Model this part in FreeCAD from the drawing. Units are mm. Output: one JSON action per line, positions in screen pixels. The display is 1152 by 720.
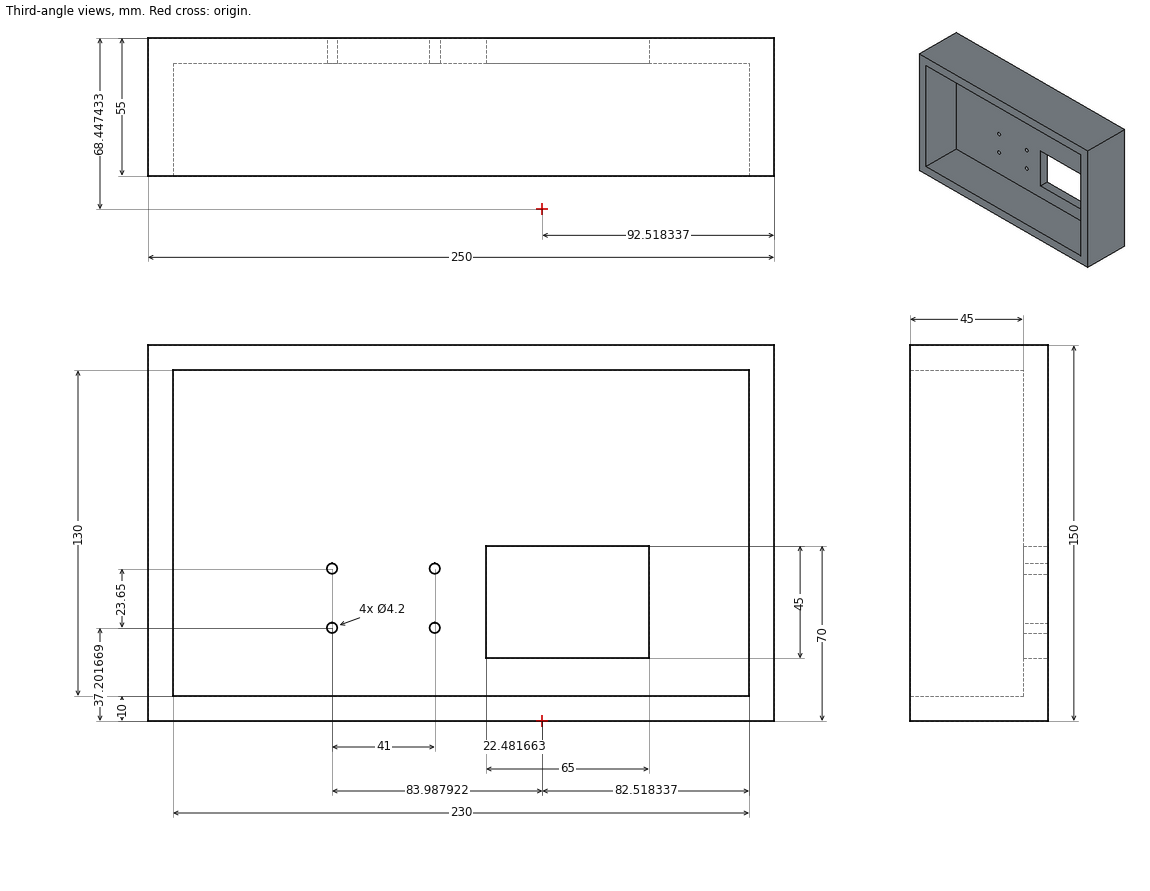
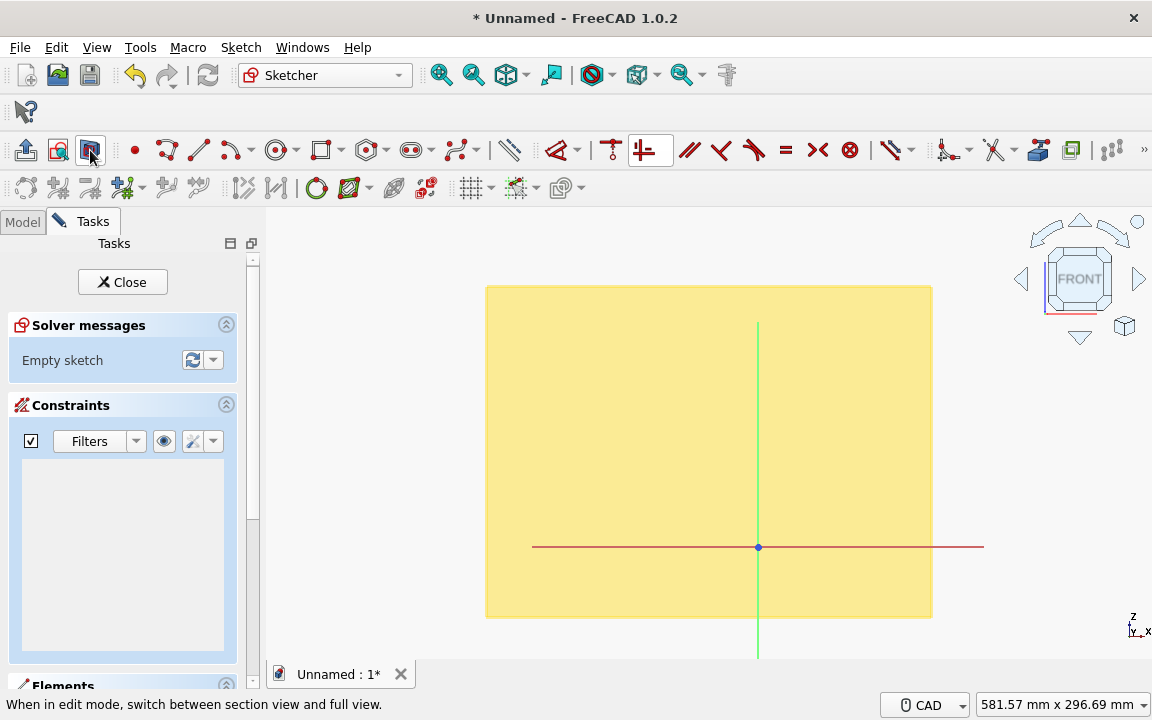
{"action": "scroll", "coordinate": [723, 538], "scroll_direction": "up", "scroll_amount": 5}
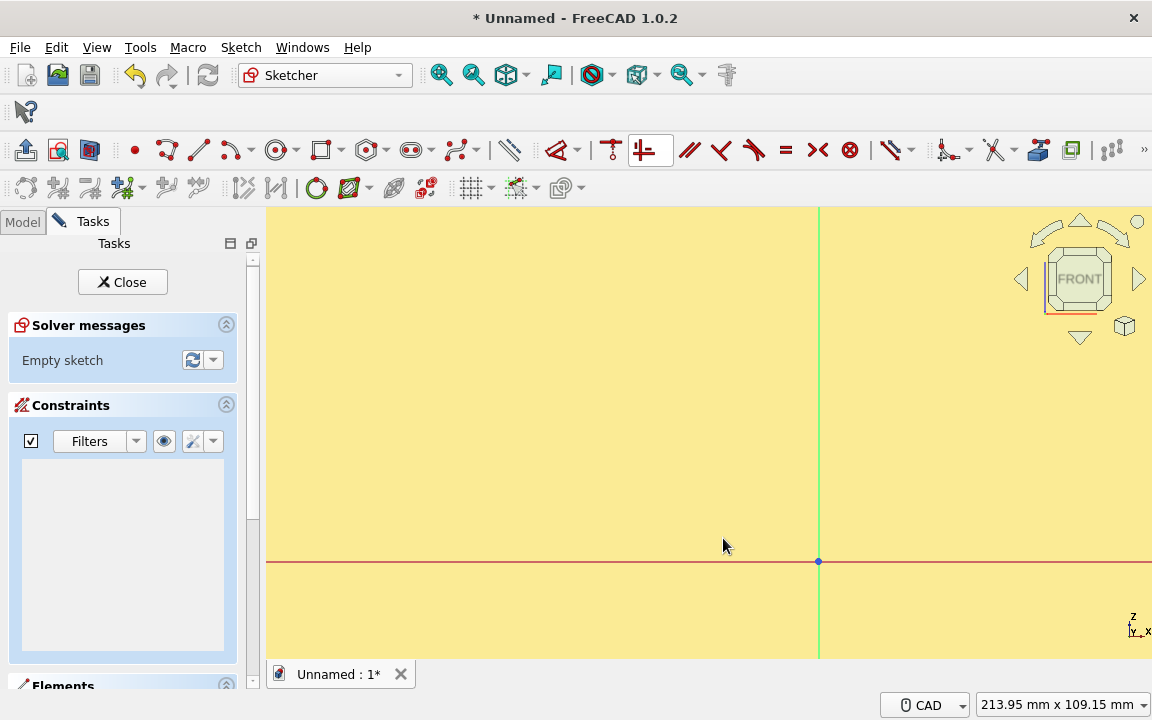
{"action": "left_click", "coordinate": [276, 150]}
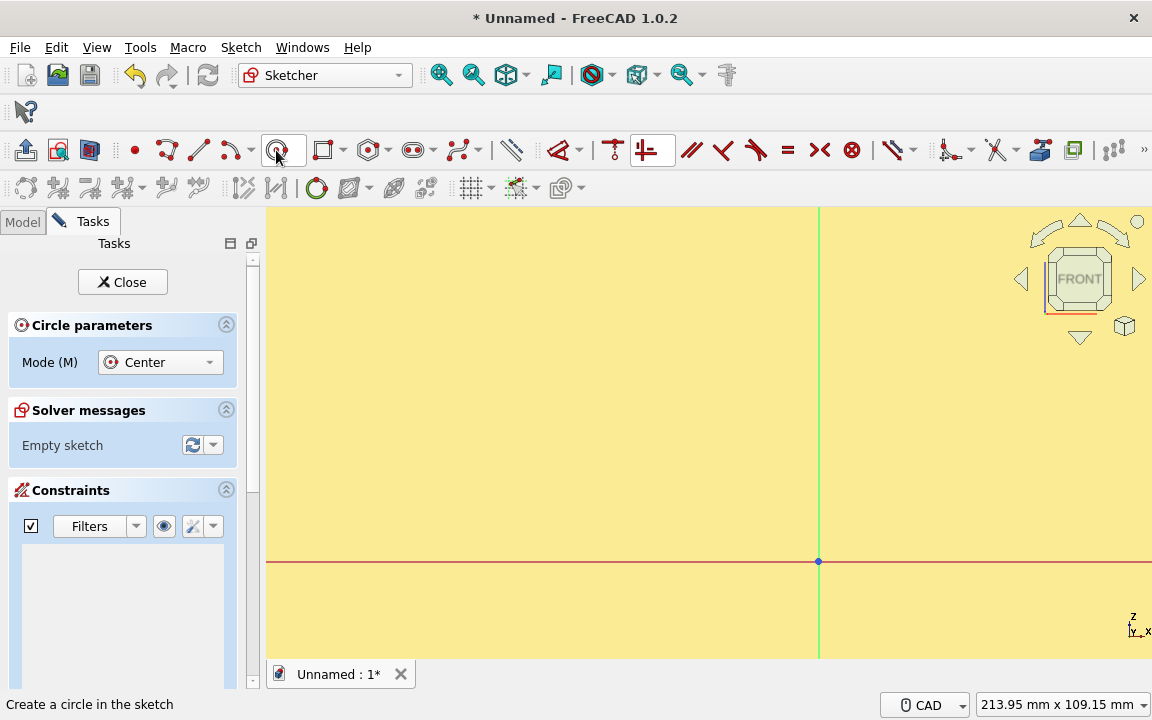
{"action": "scroll", "coordinate": [471, 408], "scroll_direction": "up", "scroll_amount": 5}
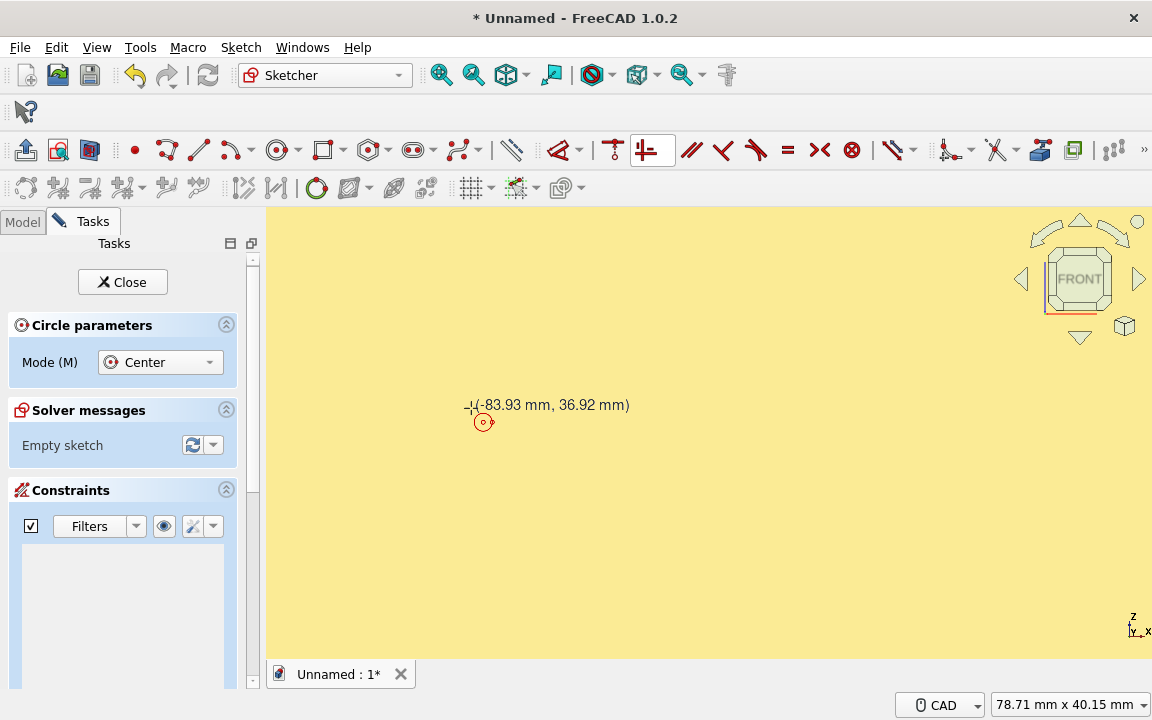
{"action": "left_click", "coordinate": [470, 407]}
{"action": "left_click", "coordinate": [487, 390]}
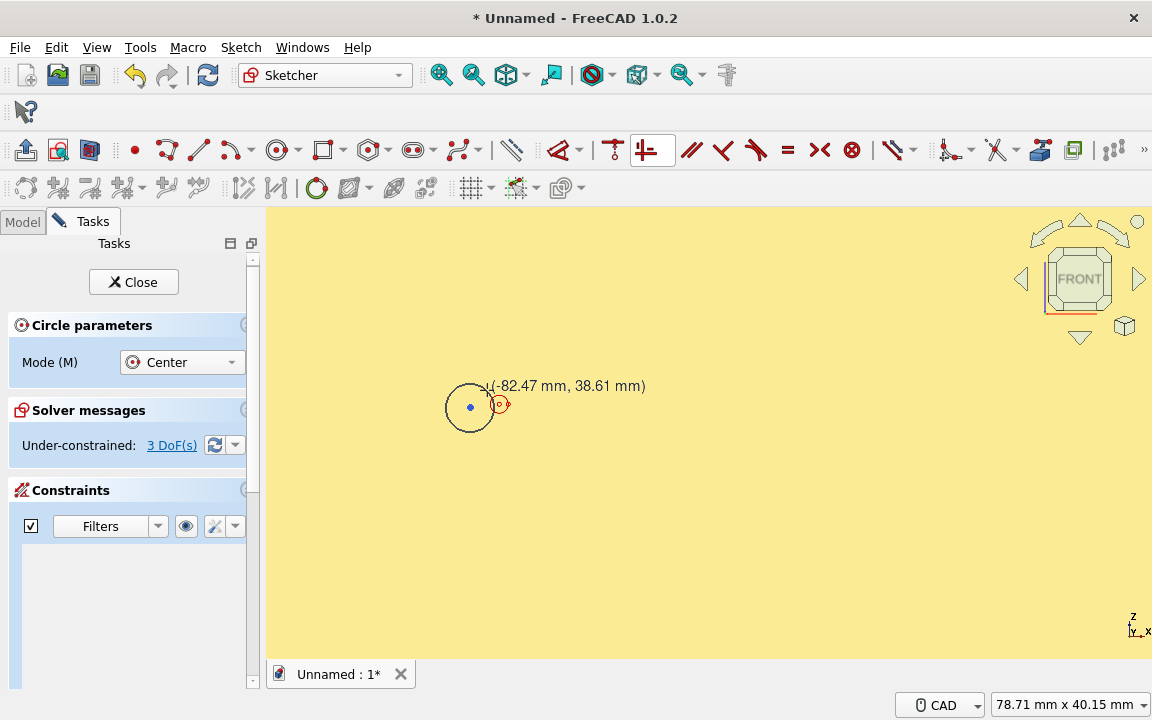
{"action": "scroll", "coordinate": [472, 411], "scroll_direction": "down", "scroll_amount": 5}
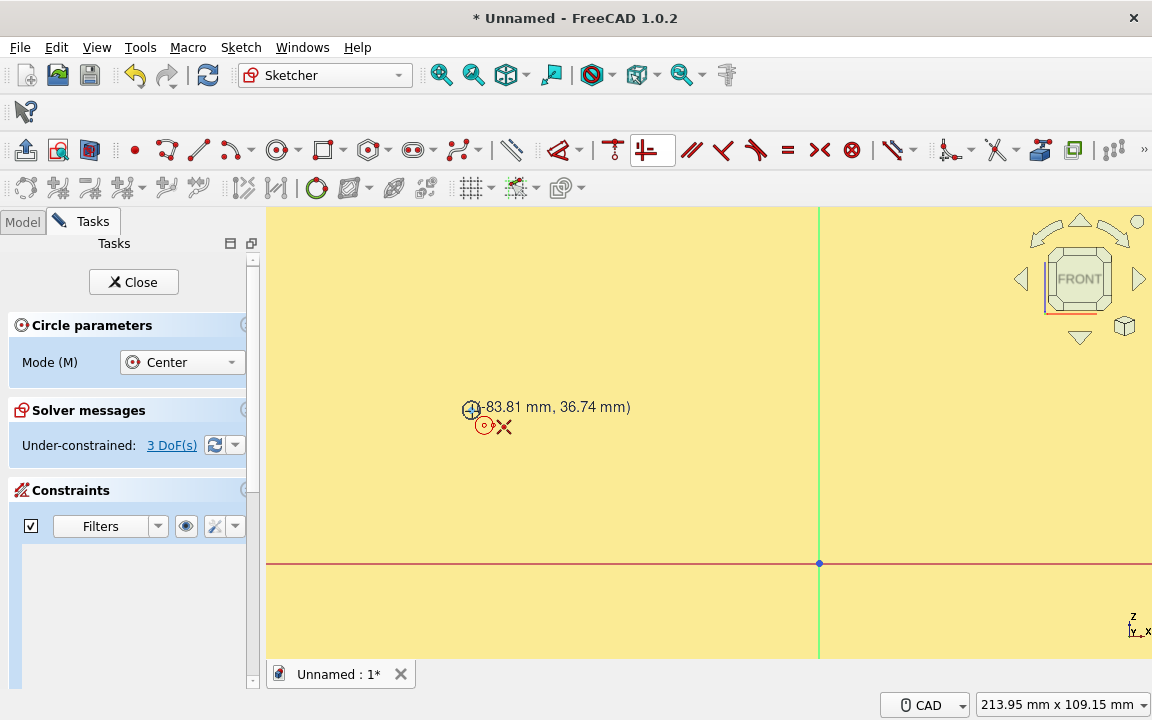
{"action": "scroll", "coordinate": [471, 312], "scroll_direction": "up", "scroll_amount": 5}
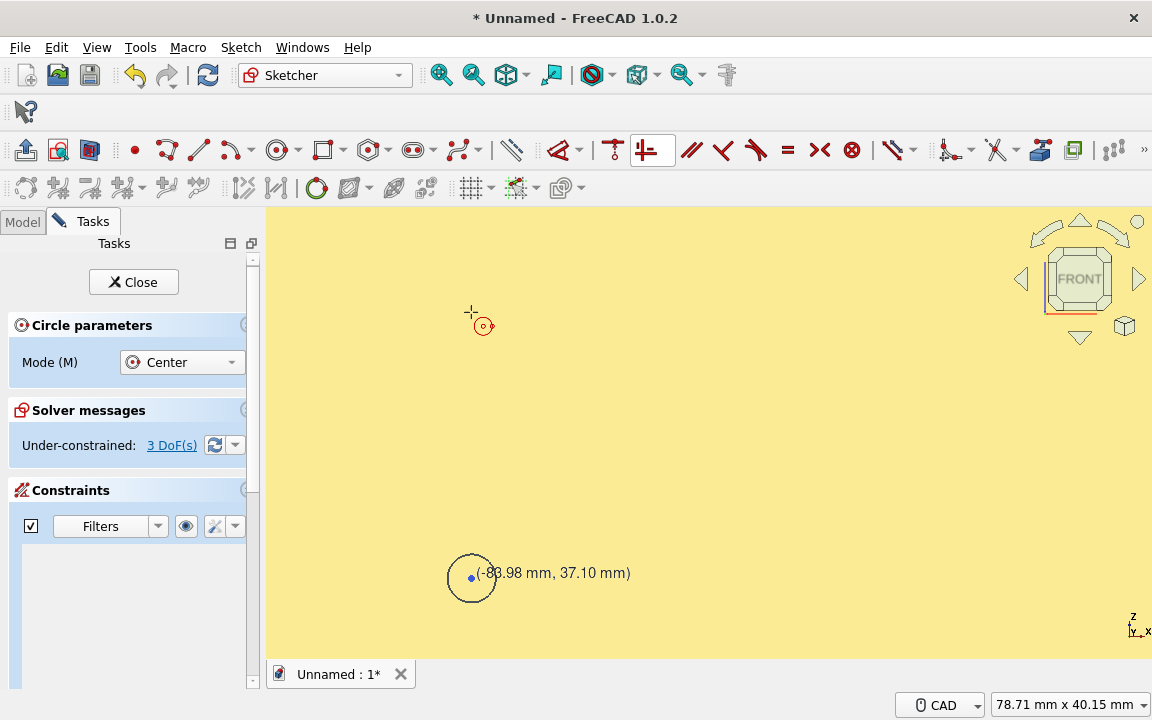
{"action": "left_click", "coordinate": [472, 311]}
{"action": "left_click", "coordinate": [488, 294]}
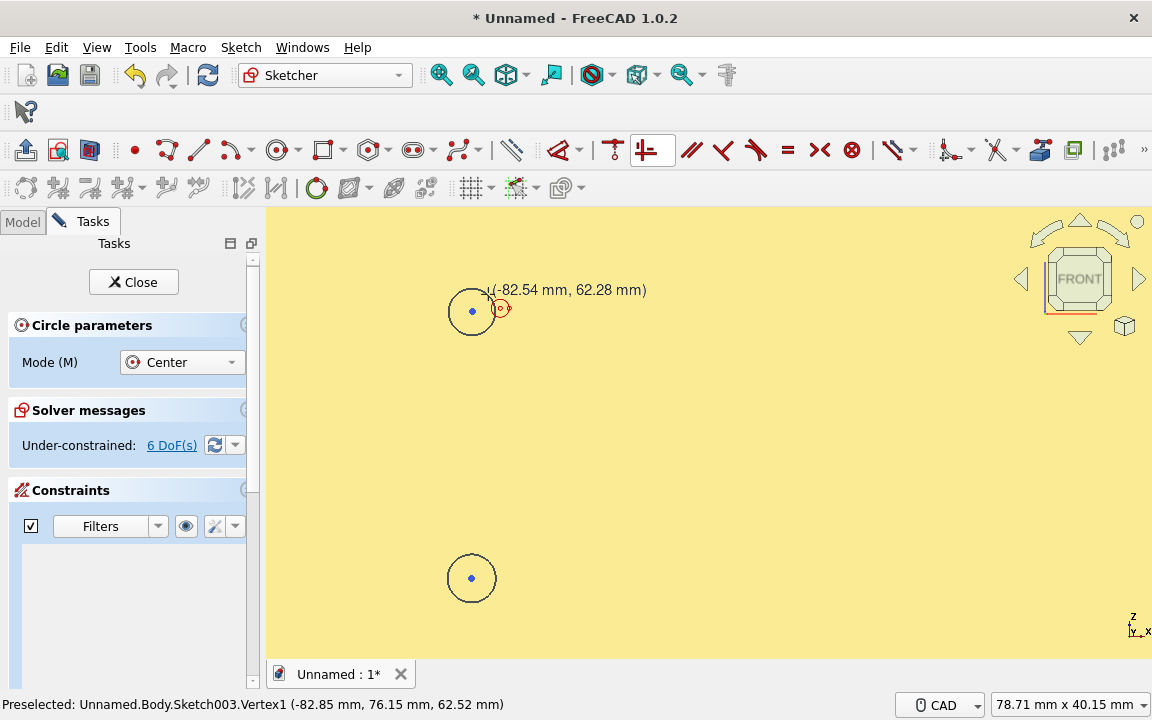
{"action": "left_click", "coordinate": [933, 311]}
{"action": "left_click", "coordinate": [950, 294]}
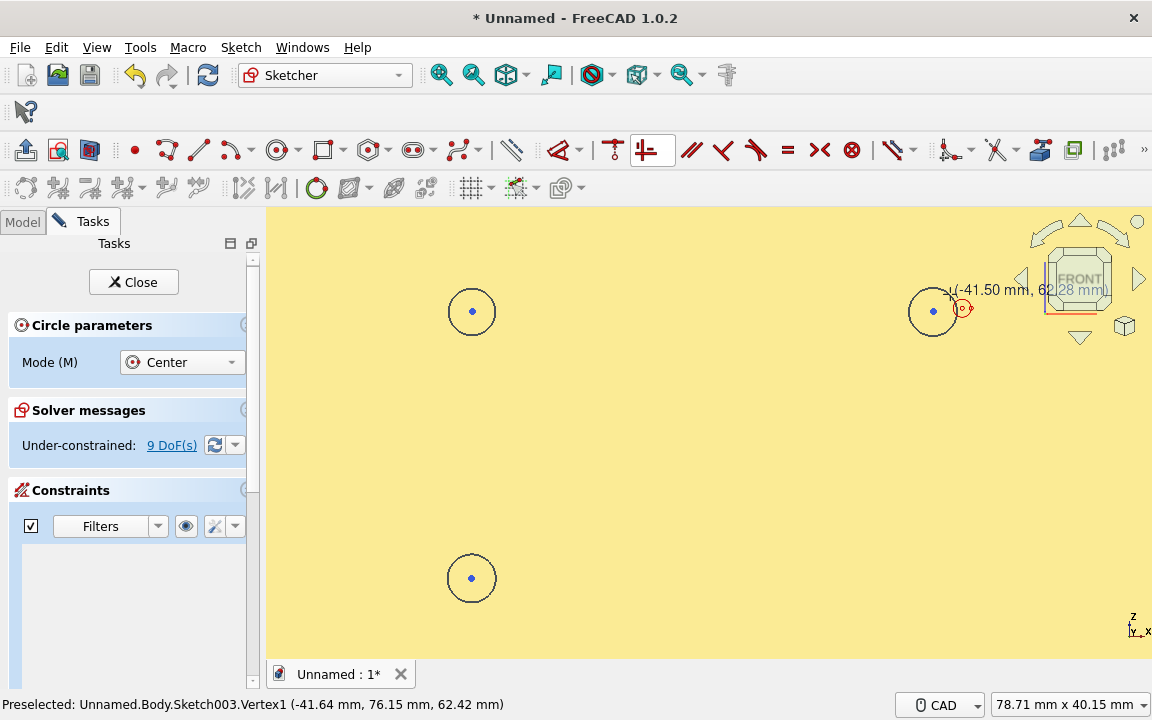
{"action": "left_click", "coordinate": [933, 577]}
{"action": "left_click", "coordinate": [950, 561]}
{"action": "key", "text": "Escape"}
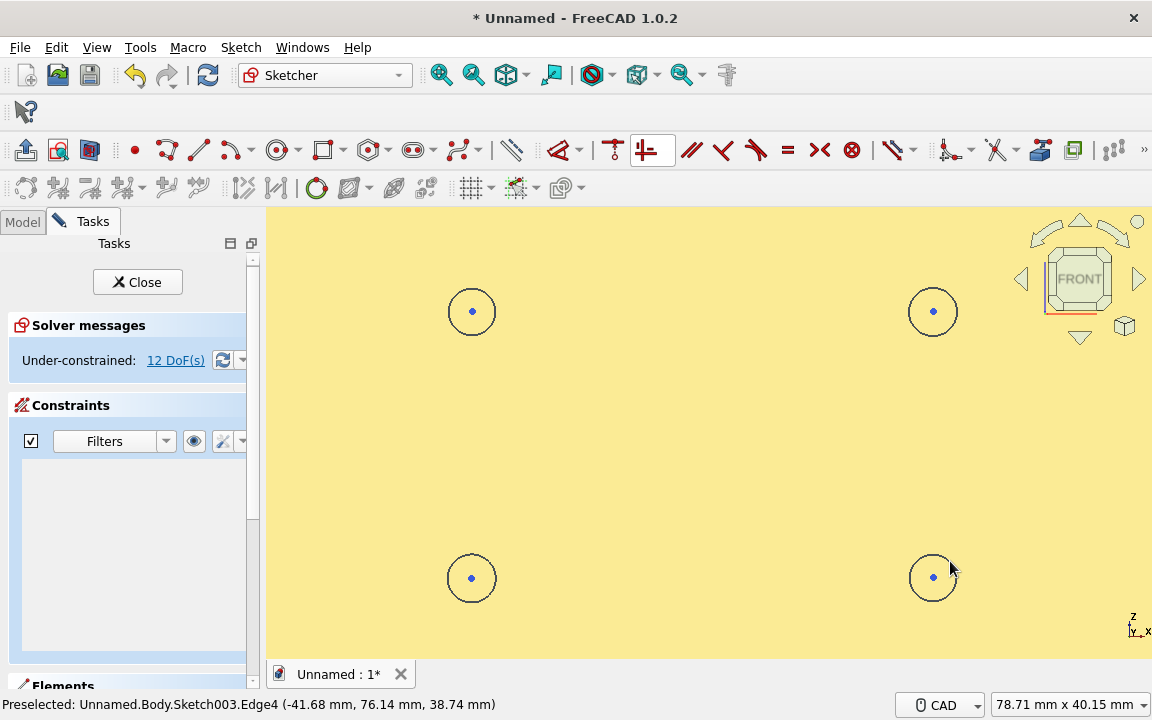
{"action": "left_click", "coordinate": [489, 561]}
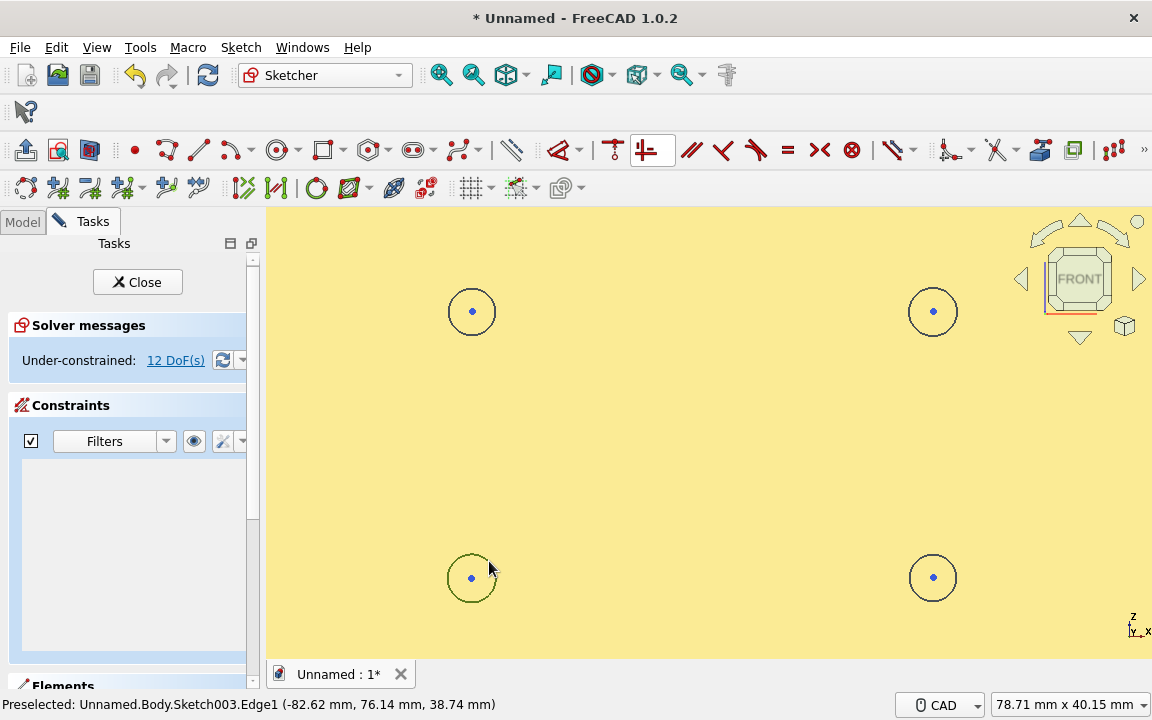
{"action": "left_click", "coordinate": [488, 295]}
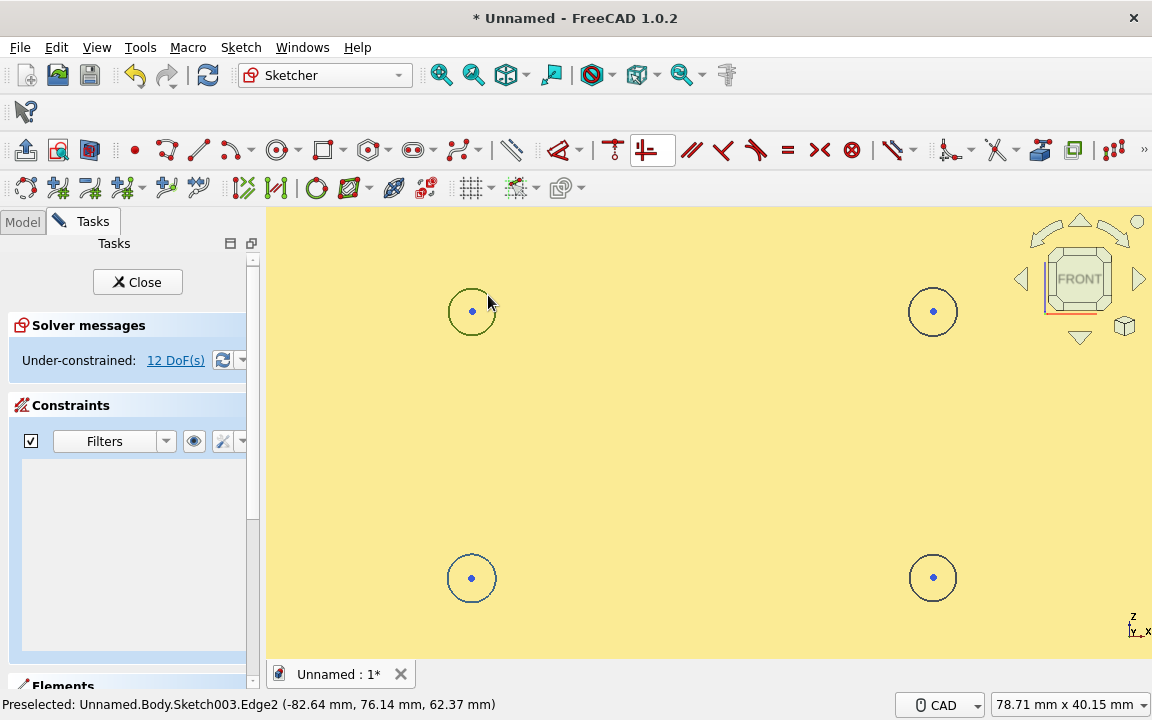
{"action": "left_click", "coordinate": [950, 295]}